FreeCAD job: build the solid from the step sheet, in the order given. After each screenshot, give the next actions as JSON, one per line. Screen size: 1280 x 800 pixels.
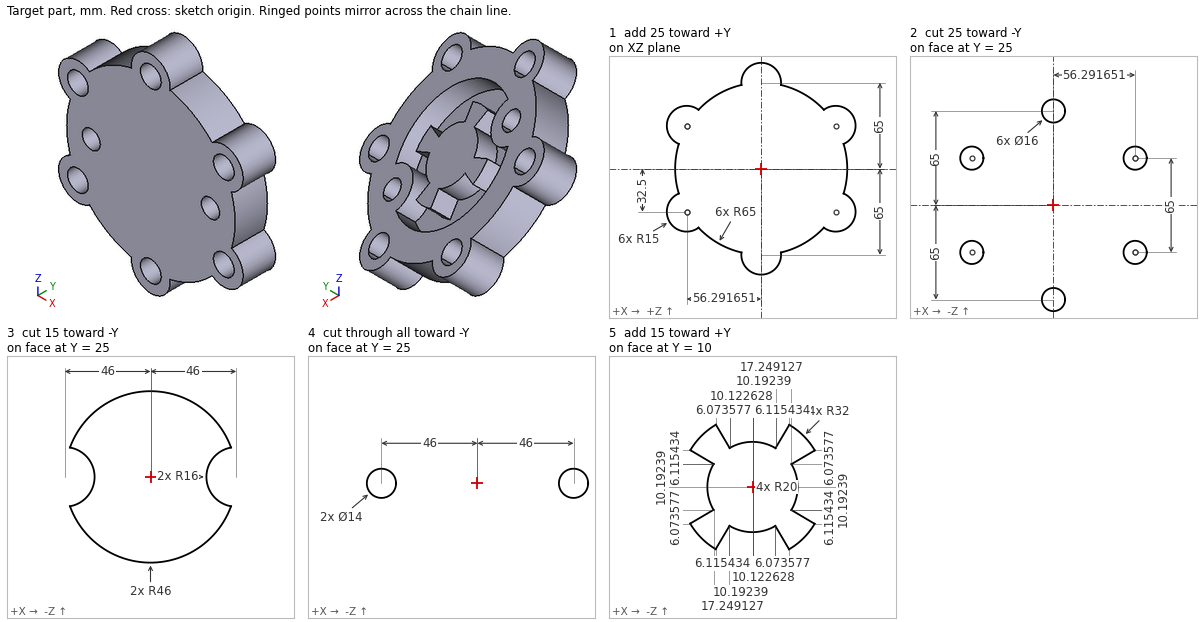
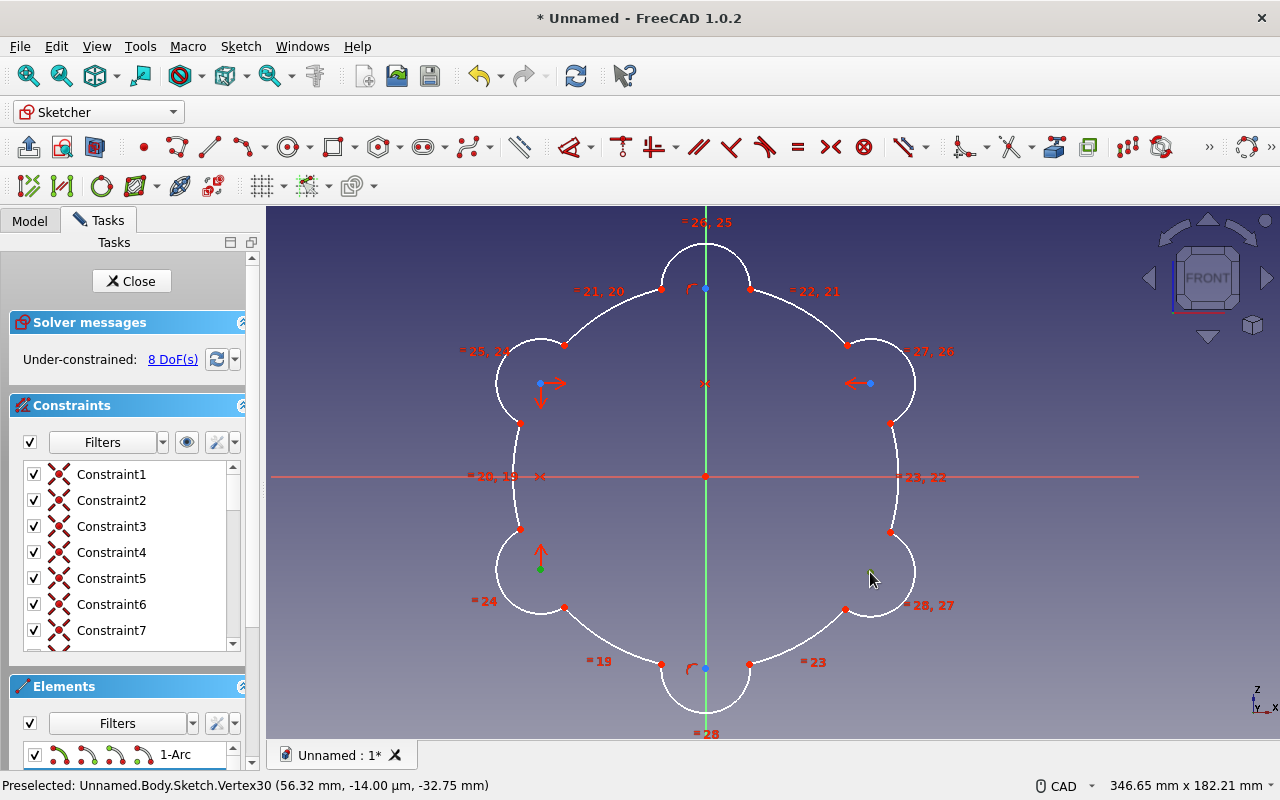
{"action": "left_click", "coordinate": [706, 677]}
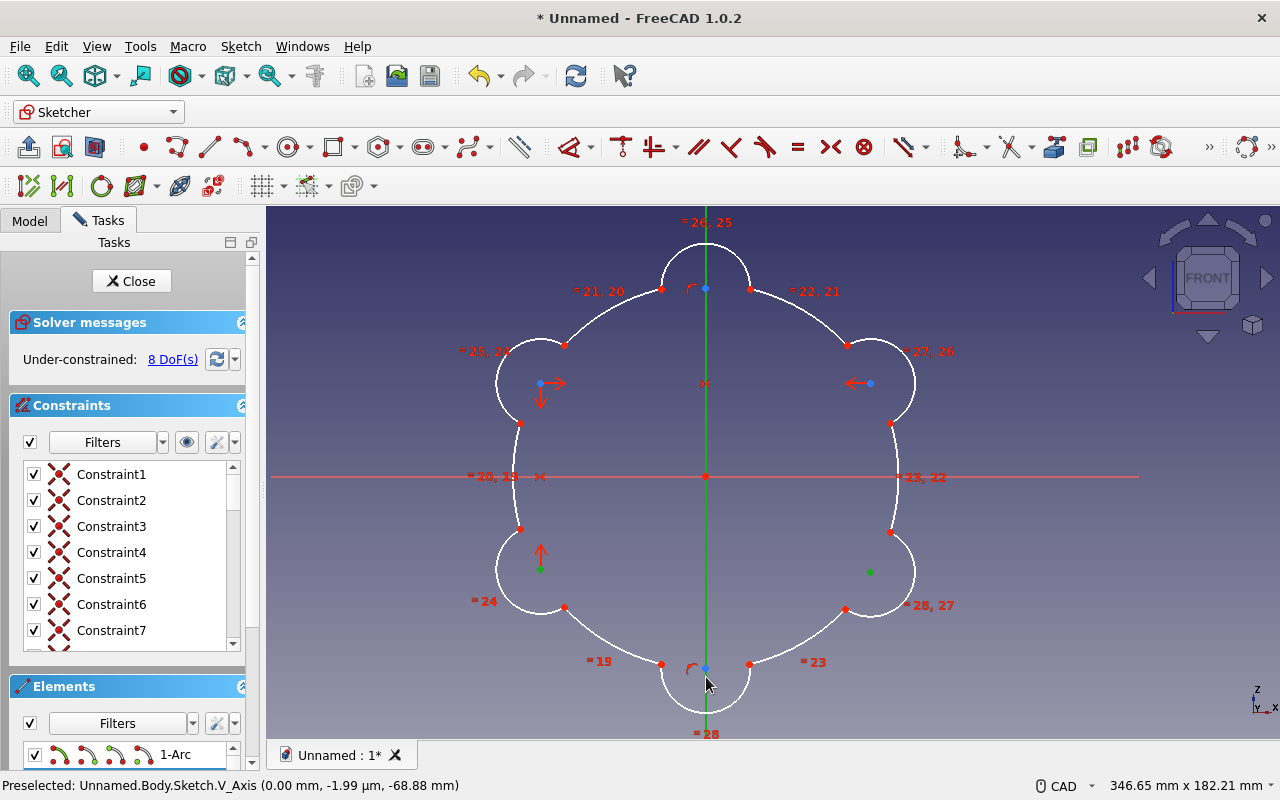
{"action": "left_click", "coordinate": [831, 148]}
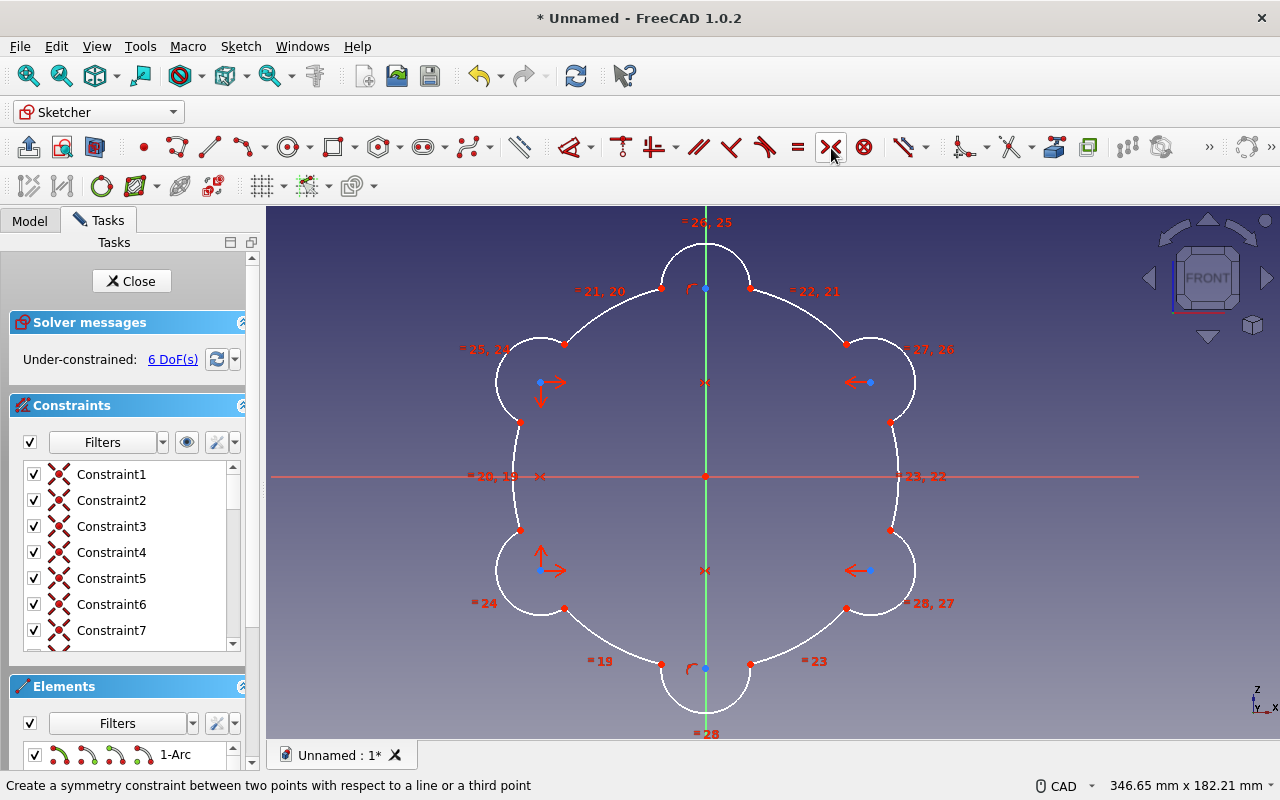
{"action": "left_click", "coordinate": [590, 631]}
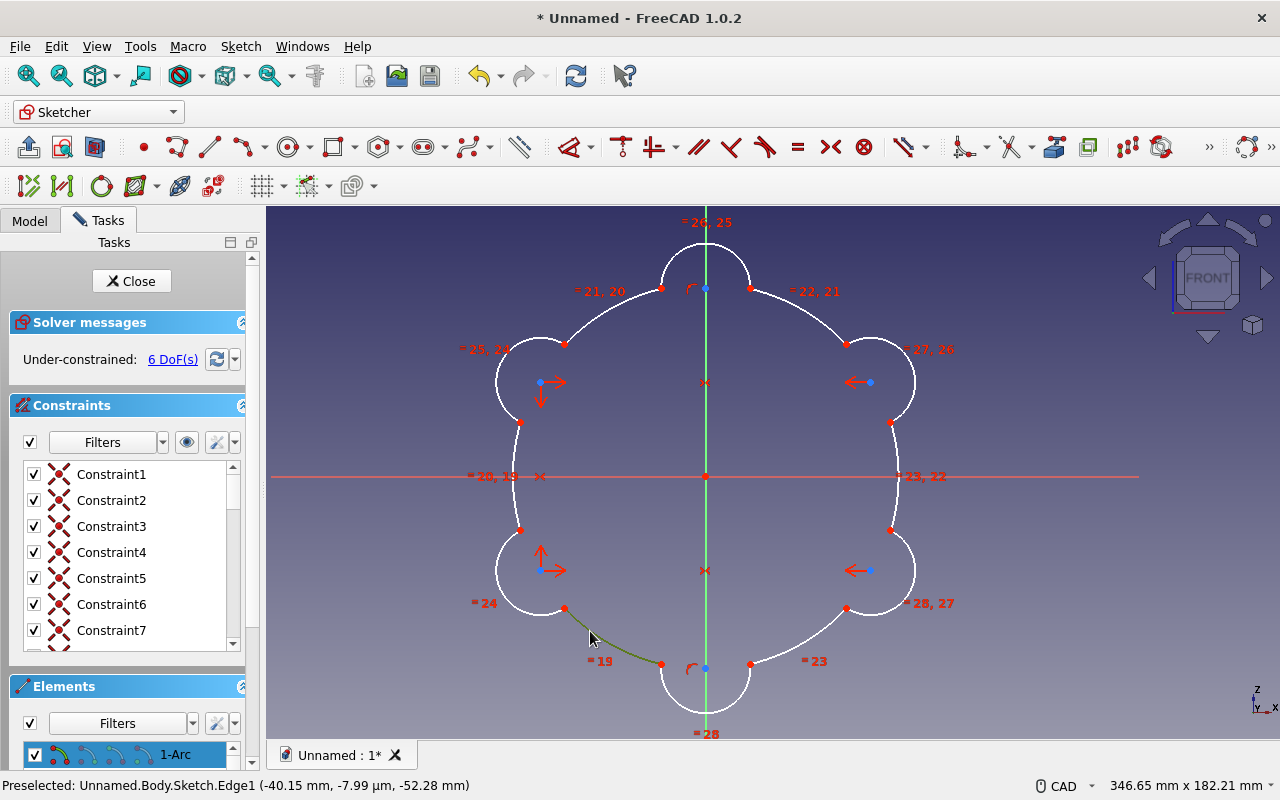
{"action": "key", "text": "k r"}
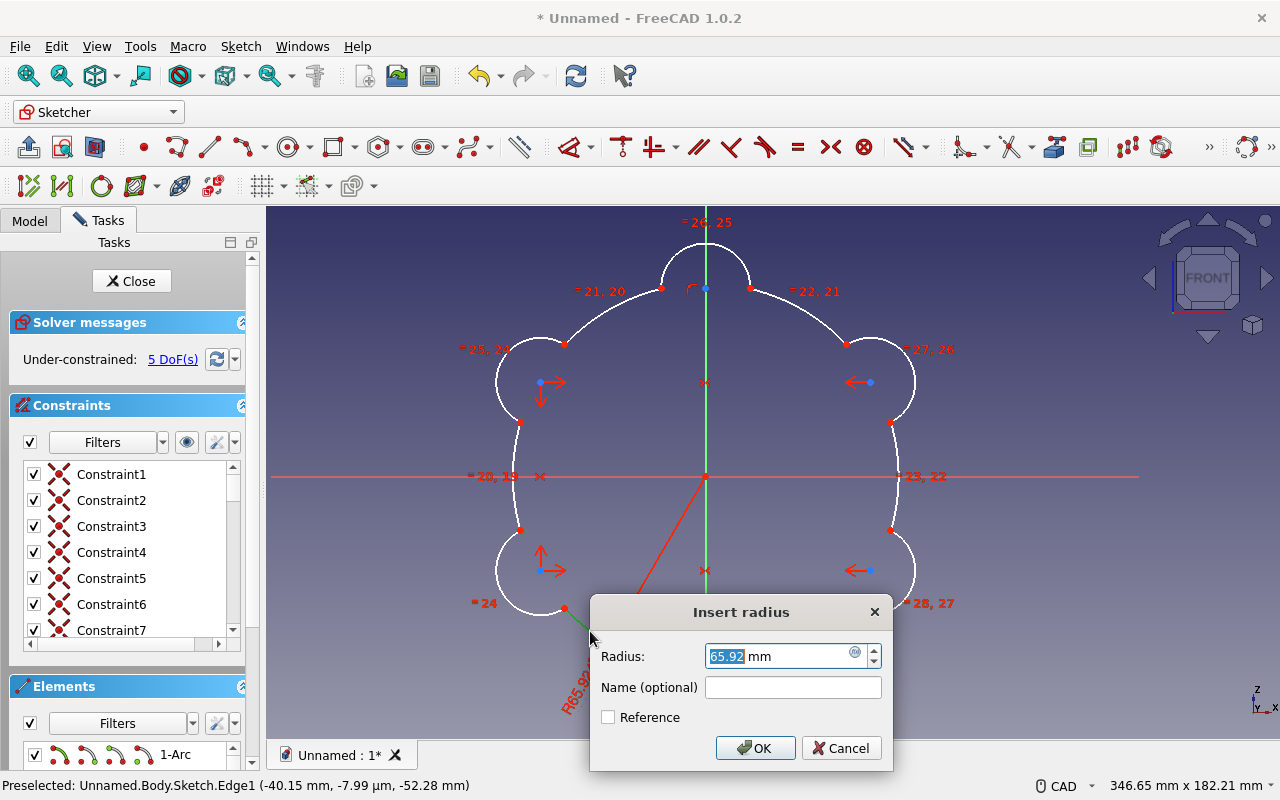
{"action": "type", "text": "65"}
{"action": "key", "text": "Return"}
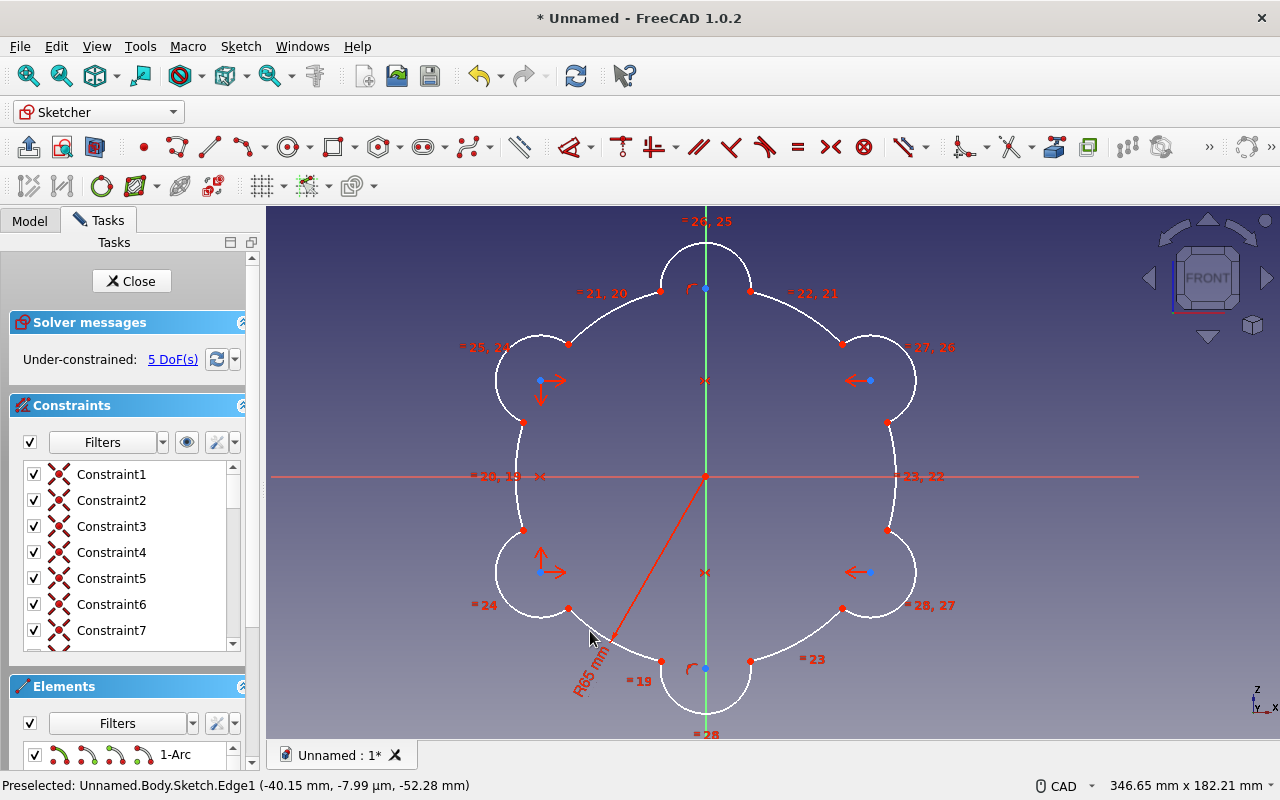
{"action": "left_click", "coordinate": [496, 565]}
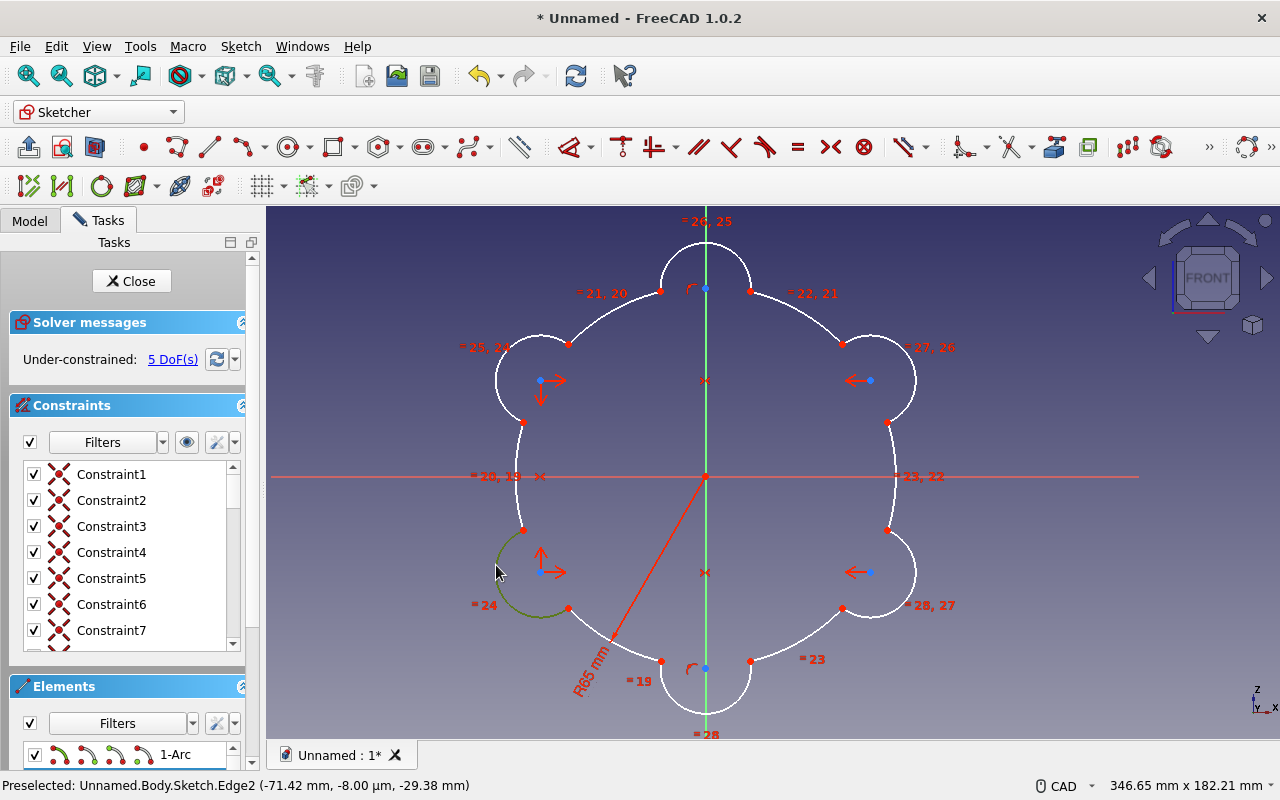
{"action": "left_click", "coordinate": [590, 148]}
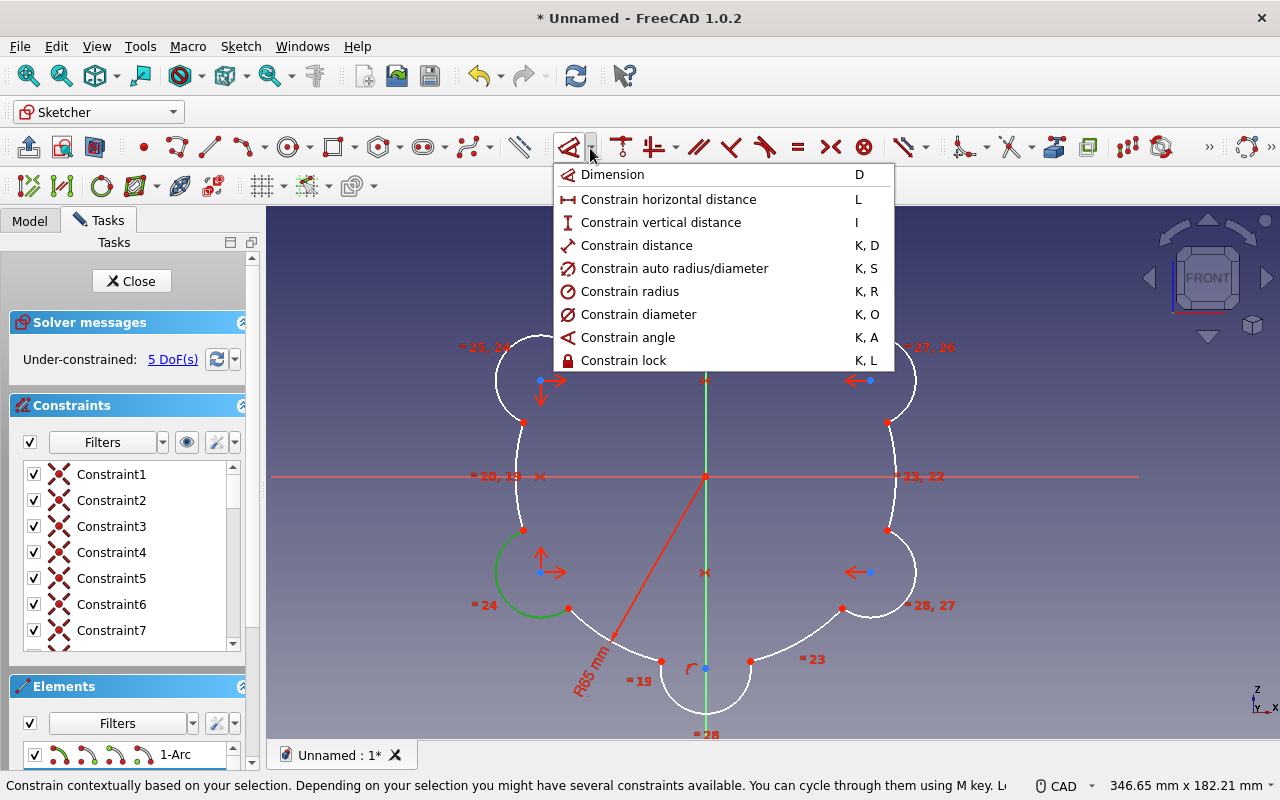
{"action": "left_click", "coordinate": [724, 292]}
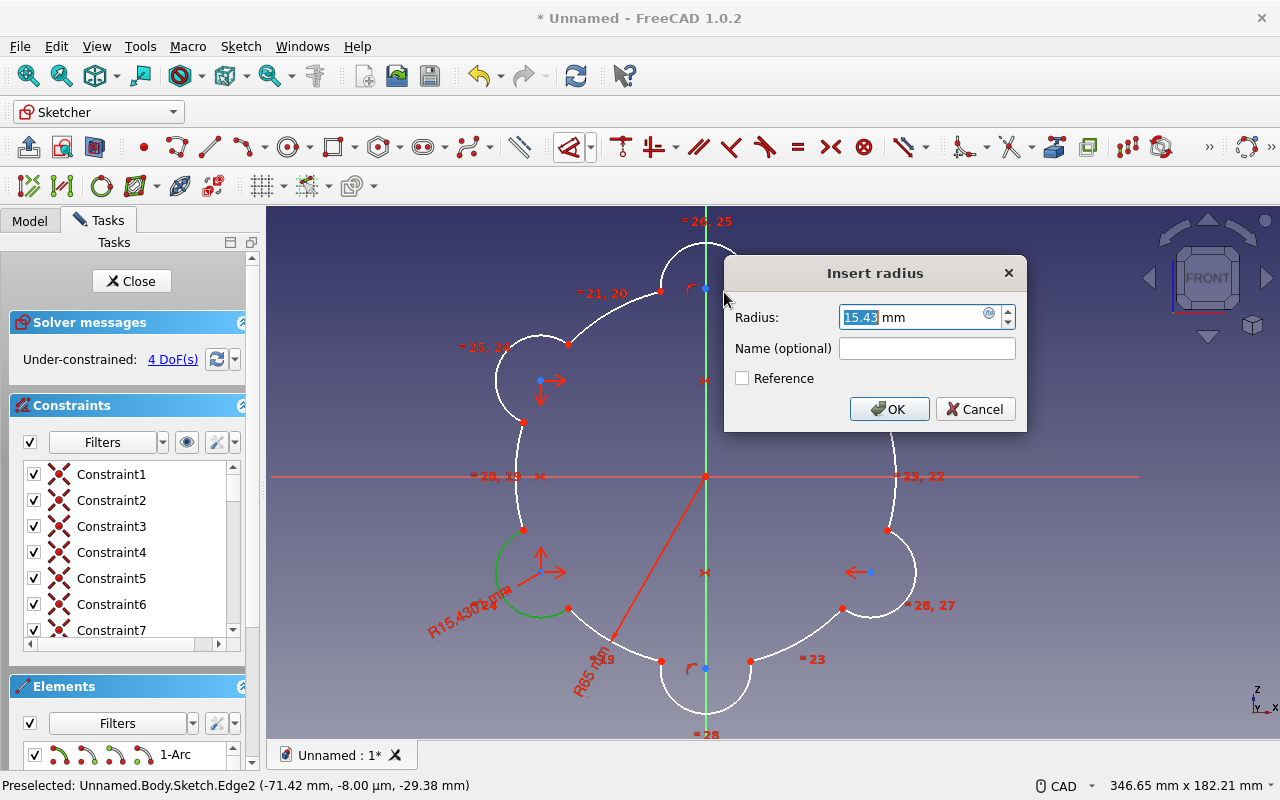
{"action": "type", "text": "15"}
{"action": "key", "text": "Return"}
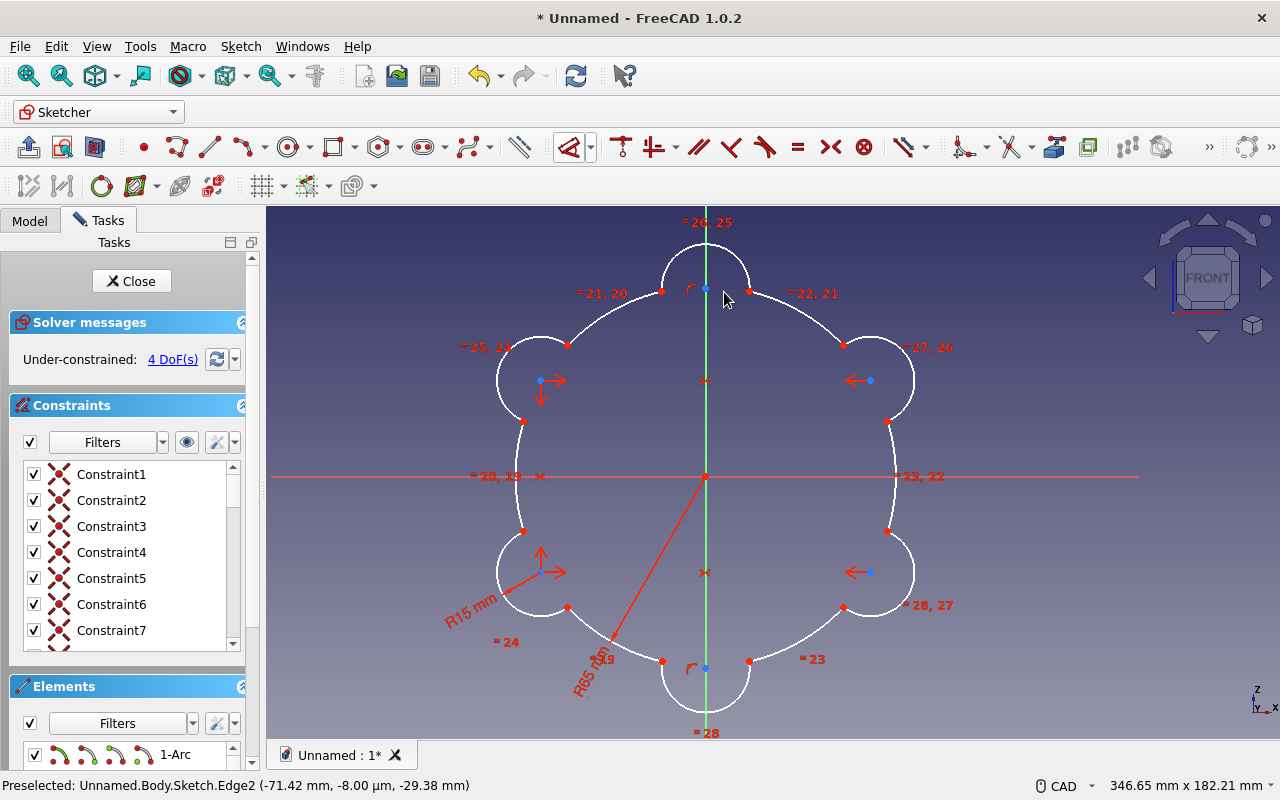
{"action": "left_click", "coordinate": [706, 288]}